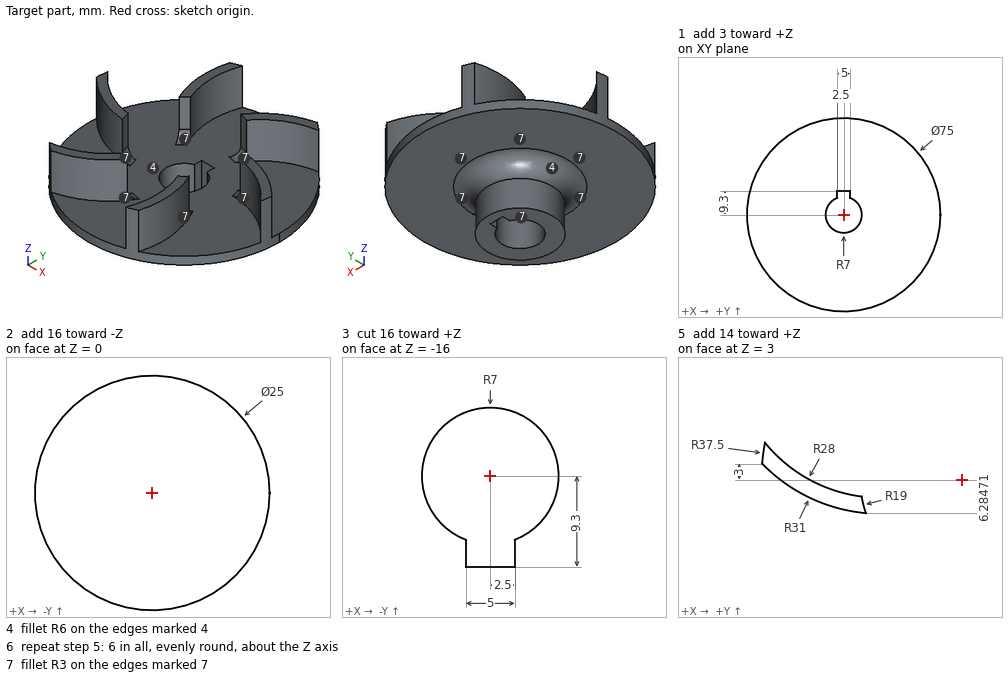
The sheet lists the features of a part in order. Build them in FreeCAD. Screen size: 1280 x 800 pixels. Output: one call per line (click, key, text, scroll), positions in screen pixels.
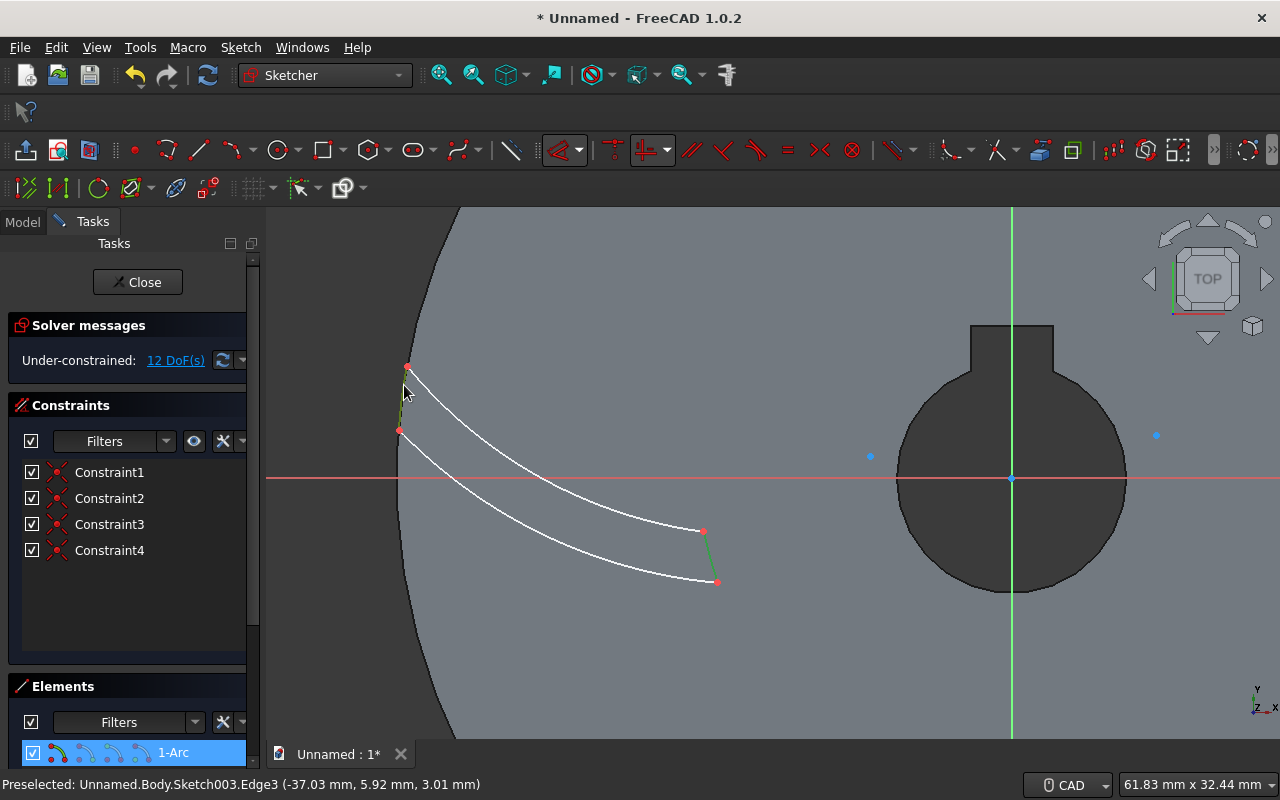
click(614, 150)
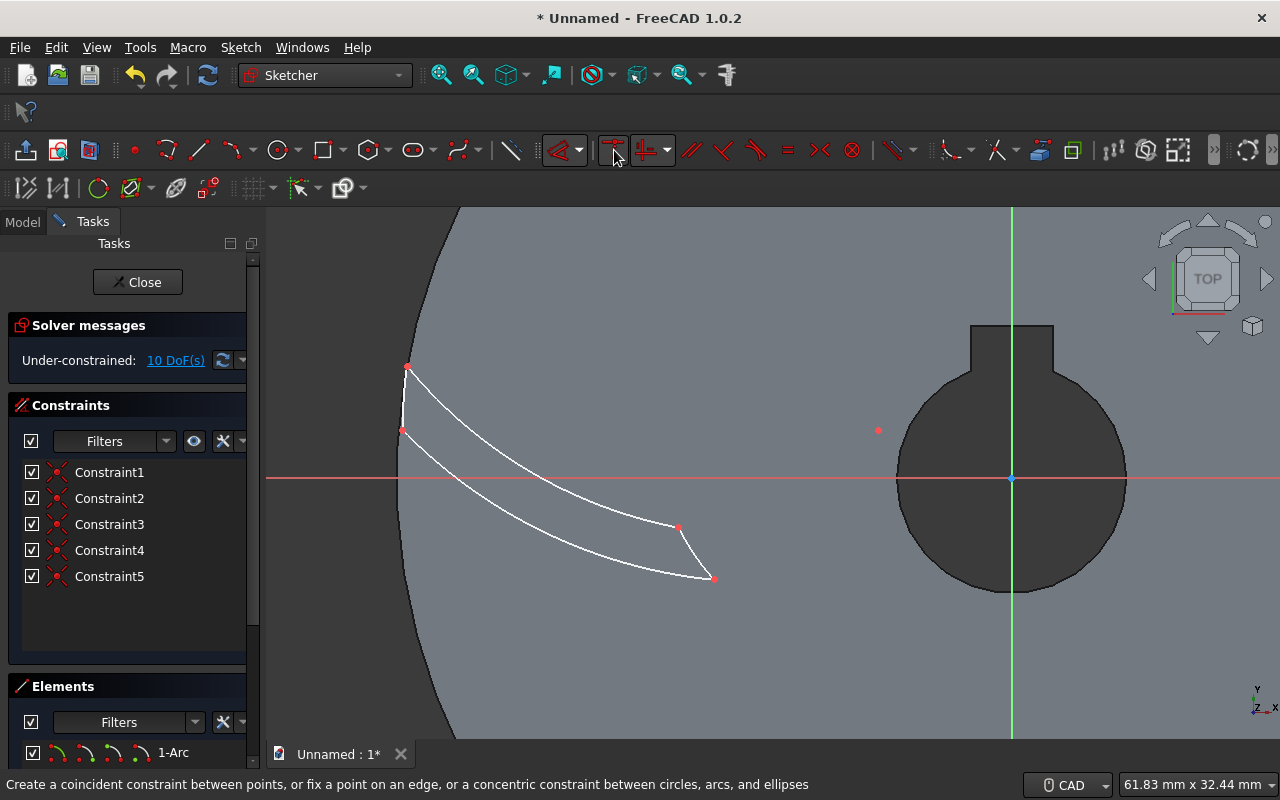
click(476, 434)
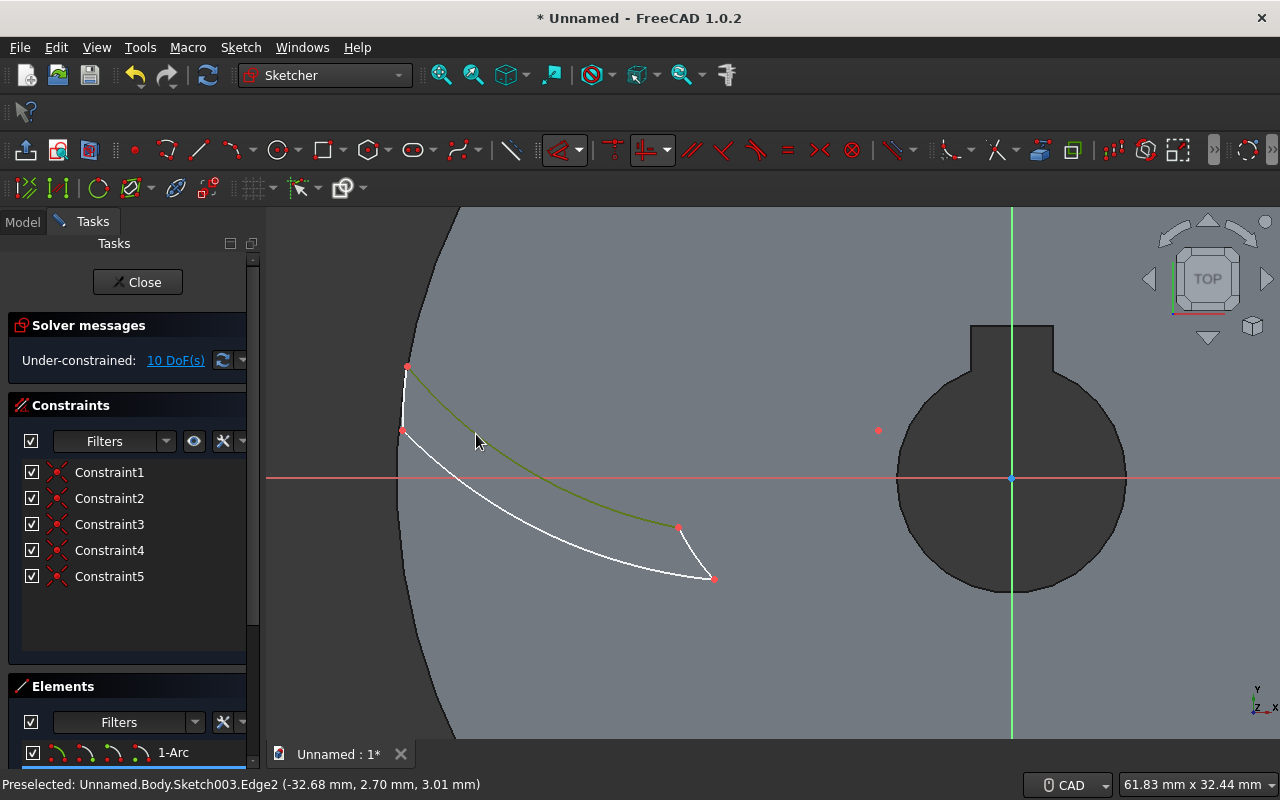
click(484, 498)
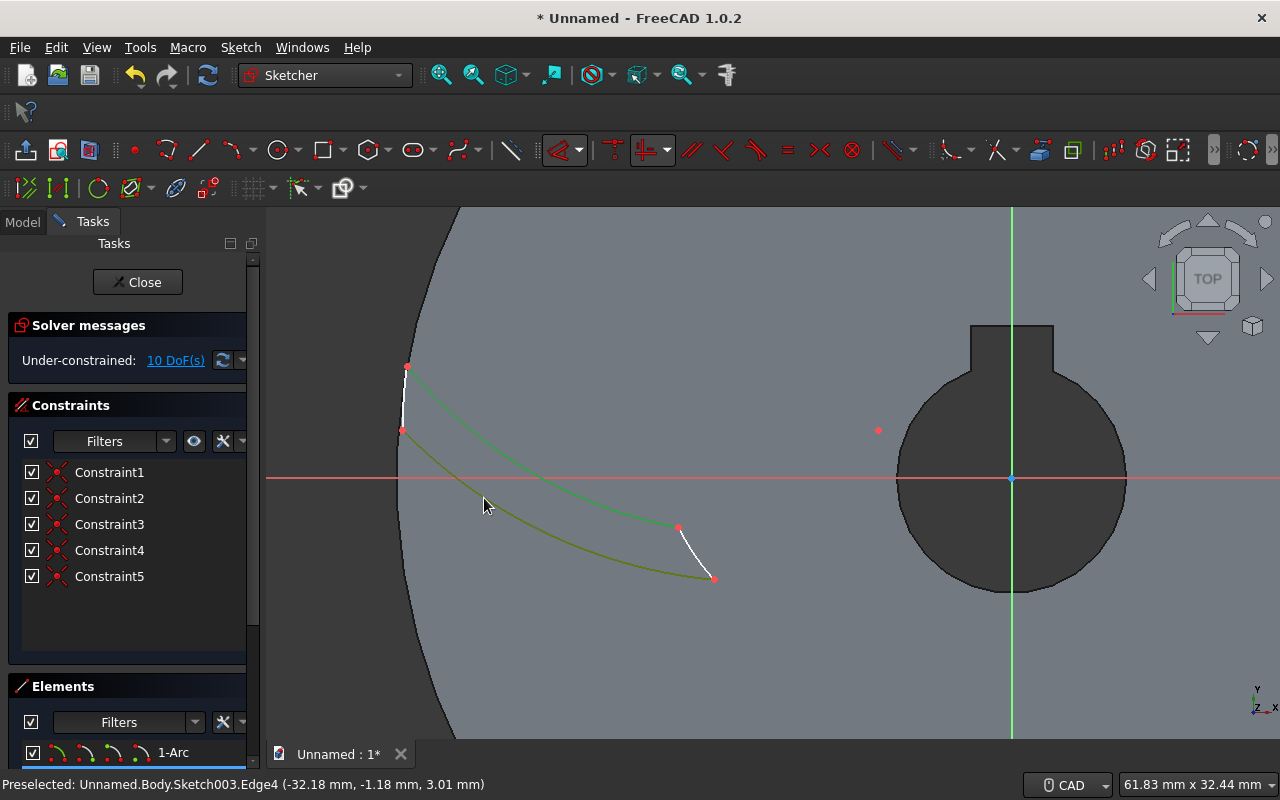
key(c)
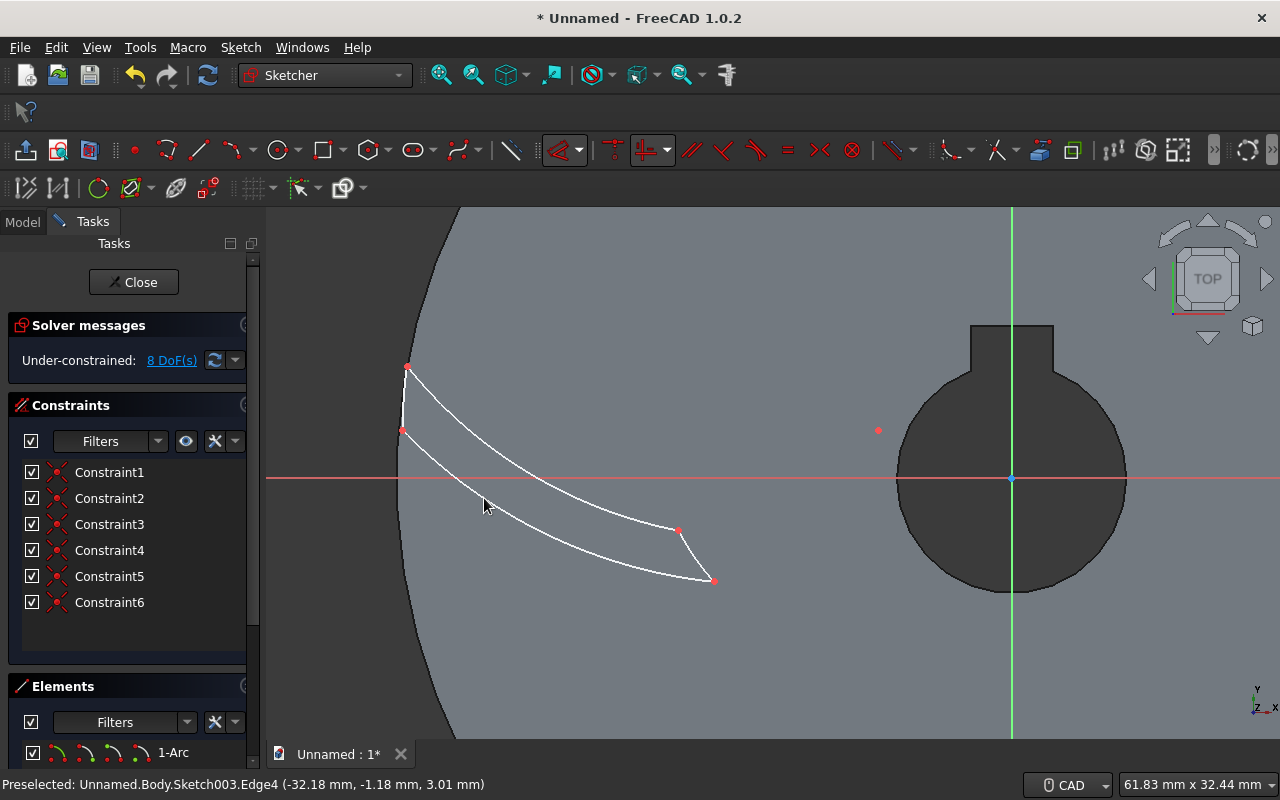
drag(869, 420, 1022, 488)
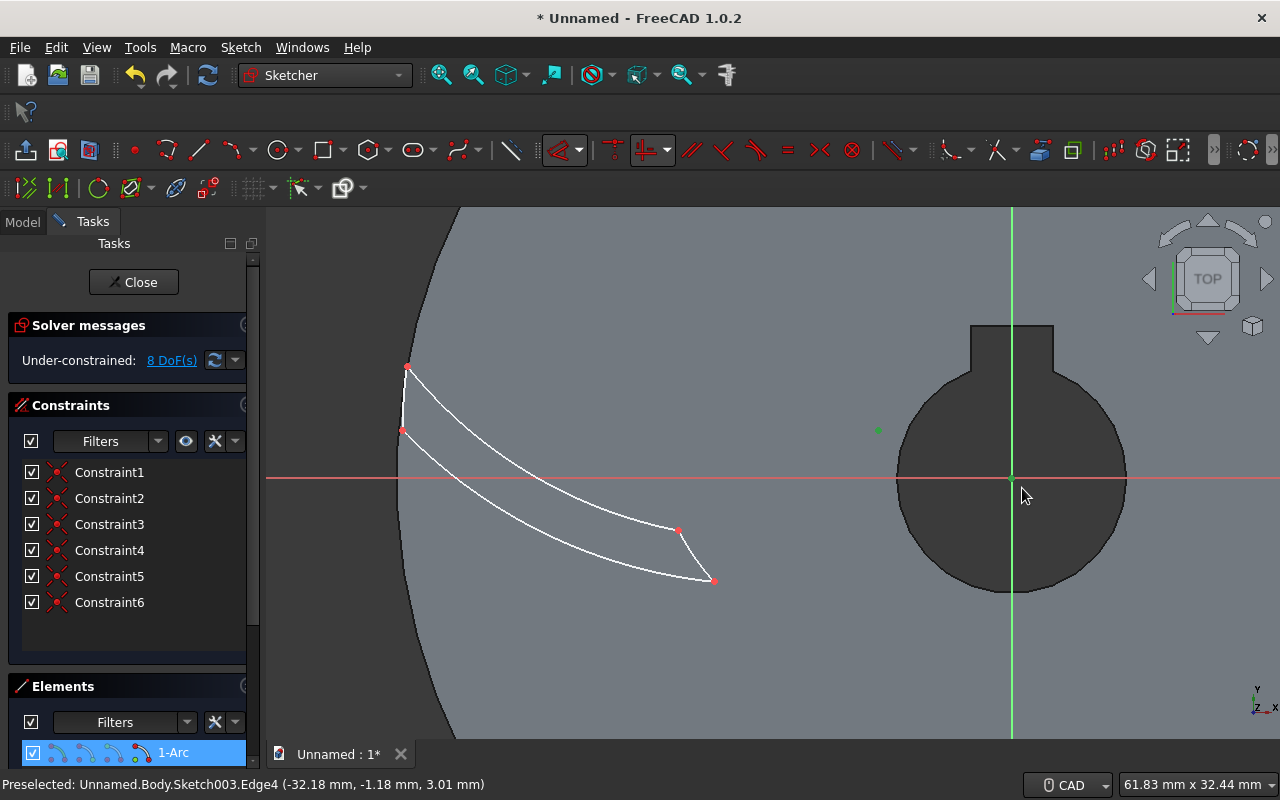
click(614, 150)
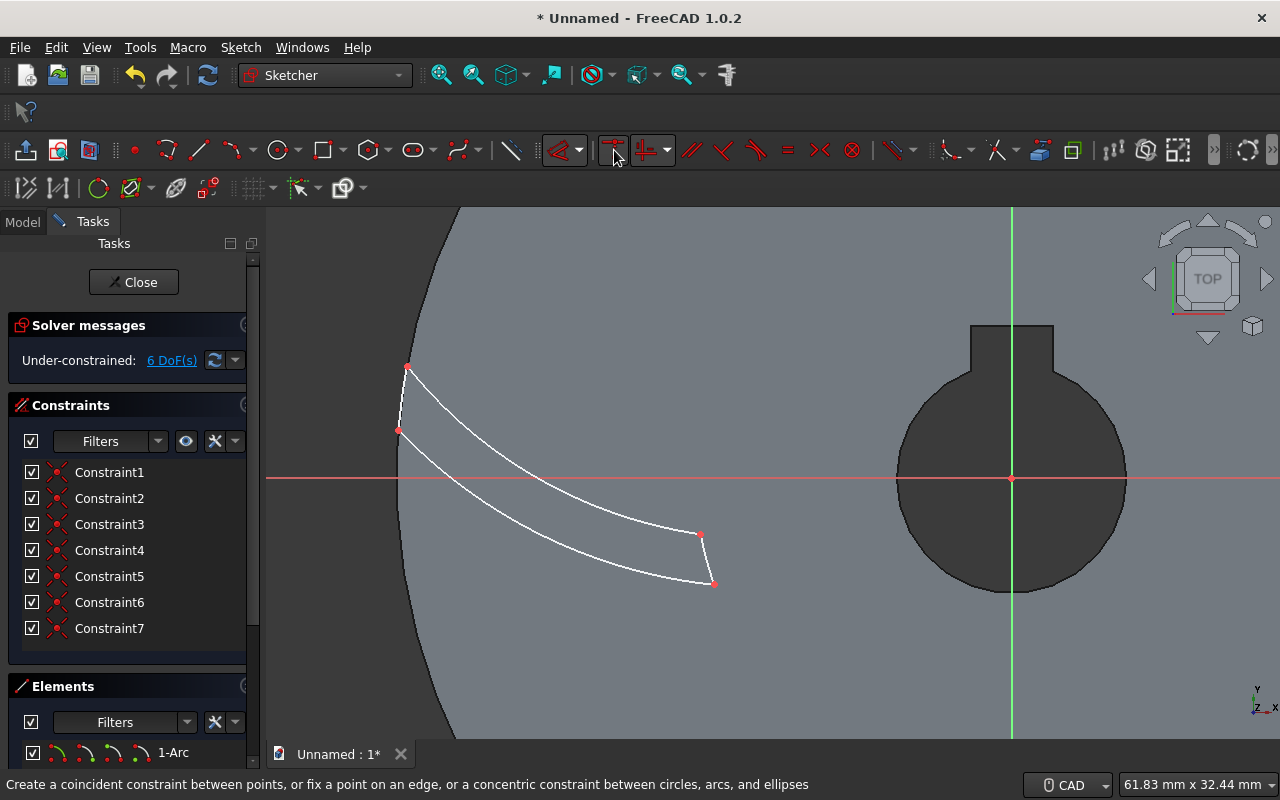
click(704, 550)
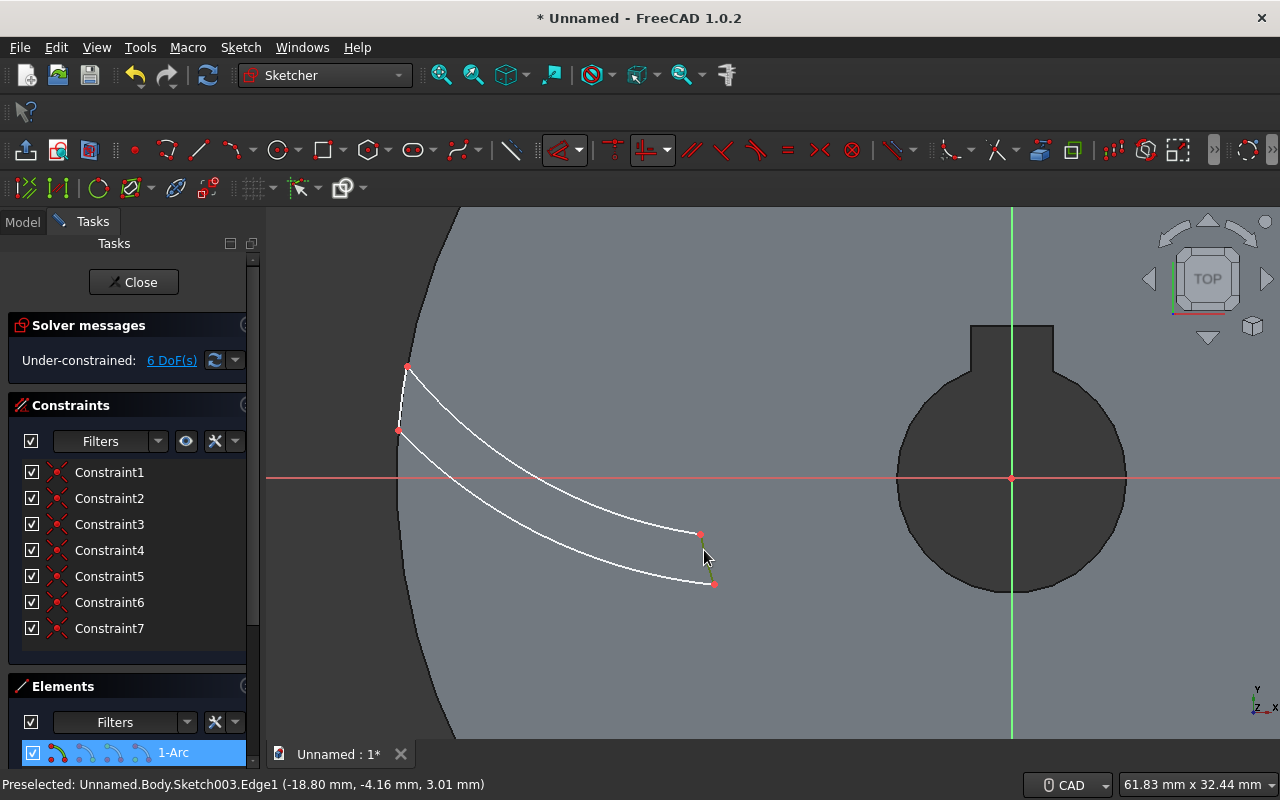
key(k)
key(r)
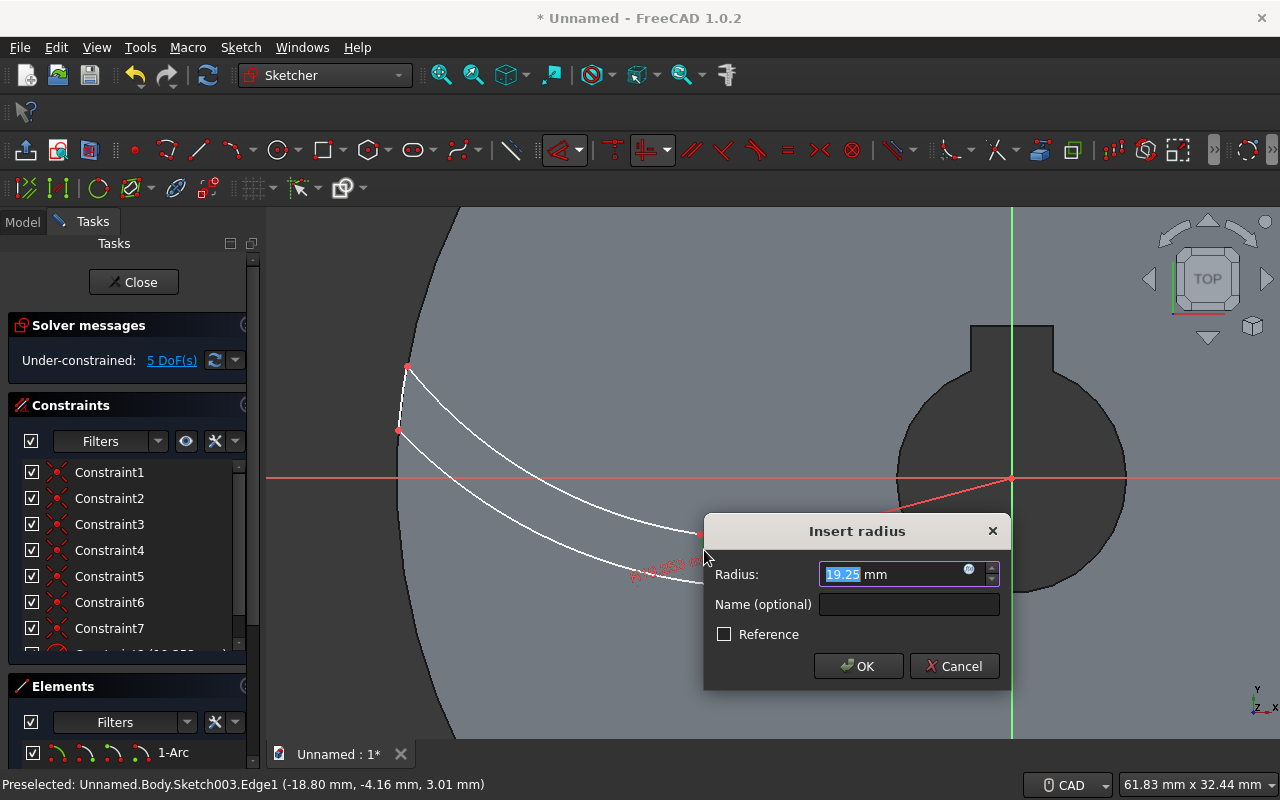
text(19)
key(Return)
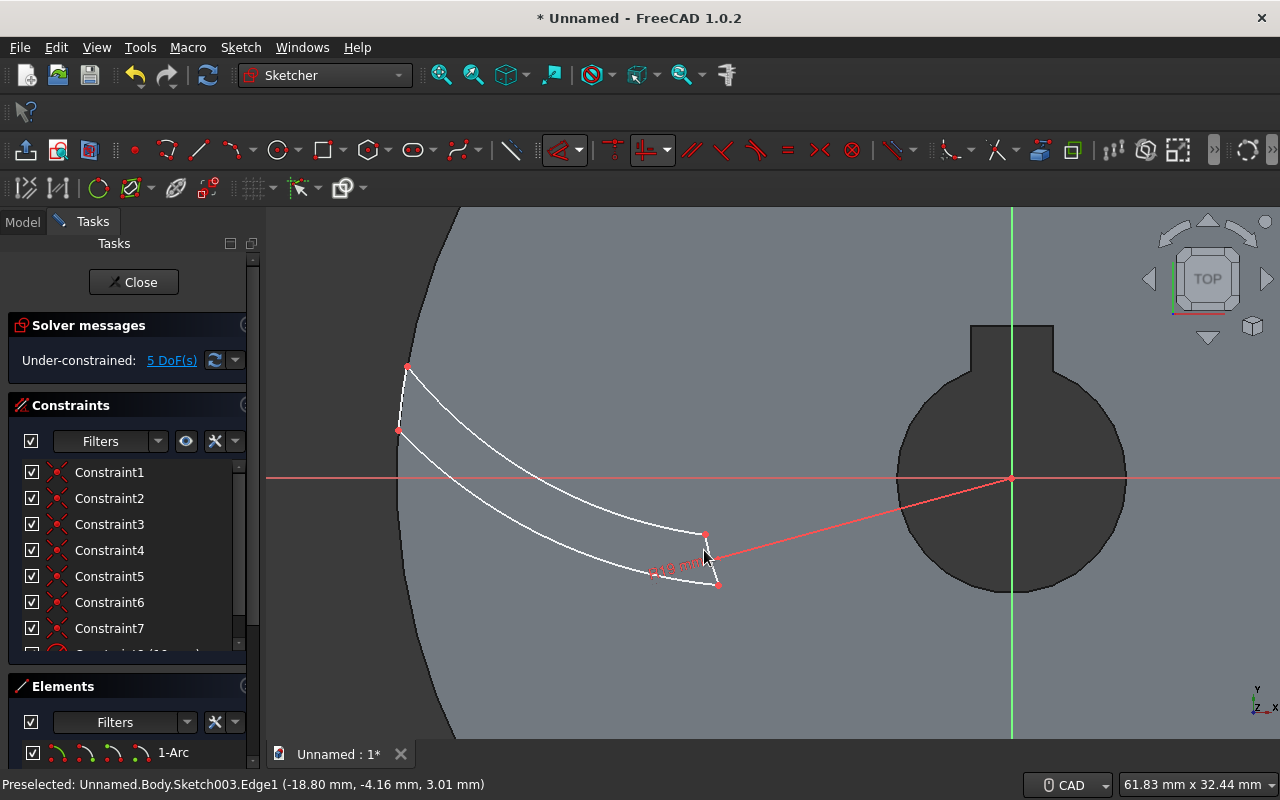
click(482, 440)